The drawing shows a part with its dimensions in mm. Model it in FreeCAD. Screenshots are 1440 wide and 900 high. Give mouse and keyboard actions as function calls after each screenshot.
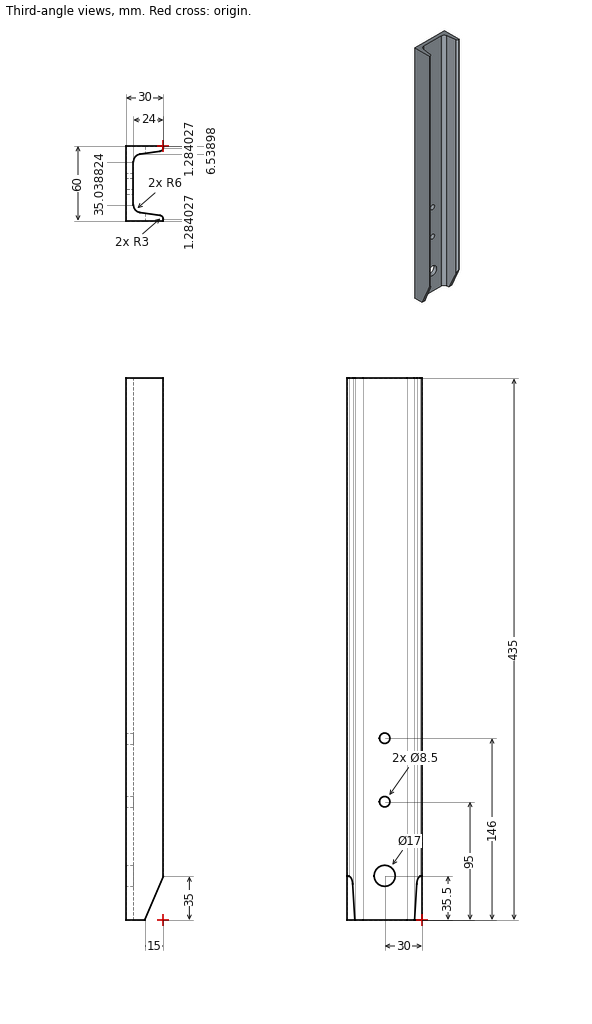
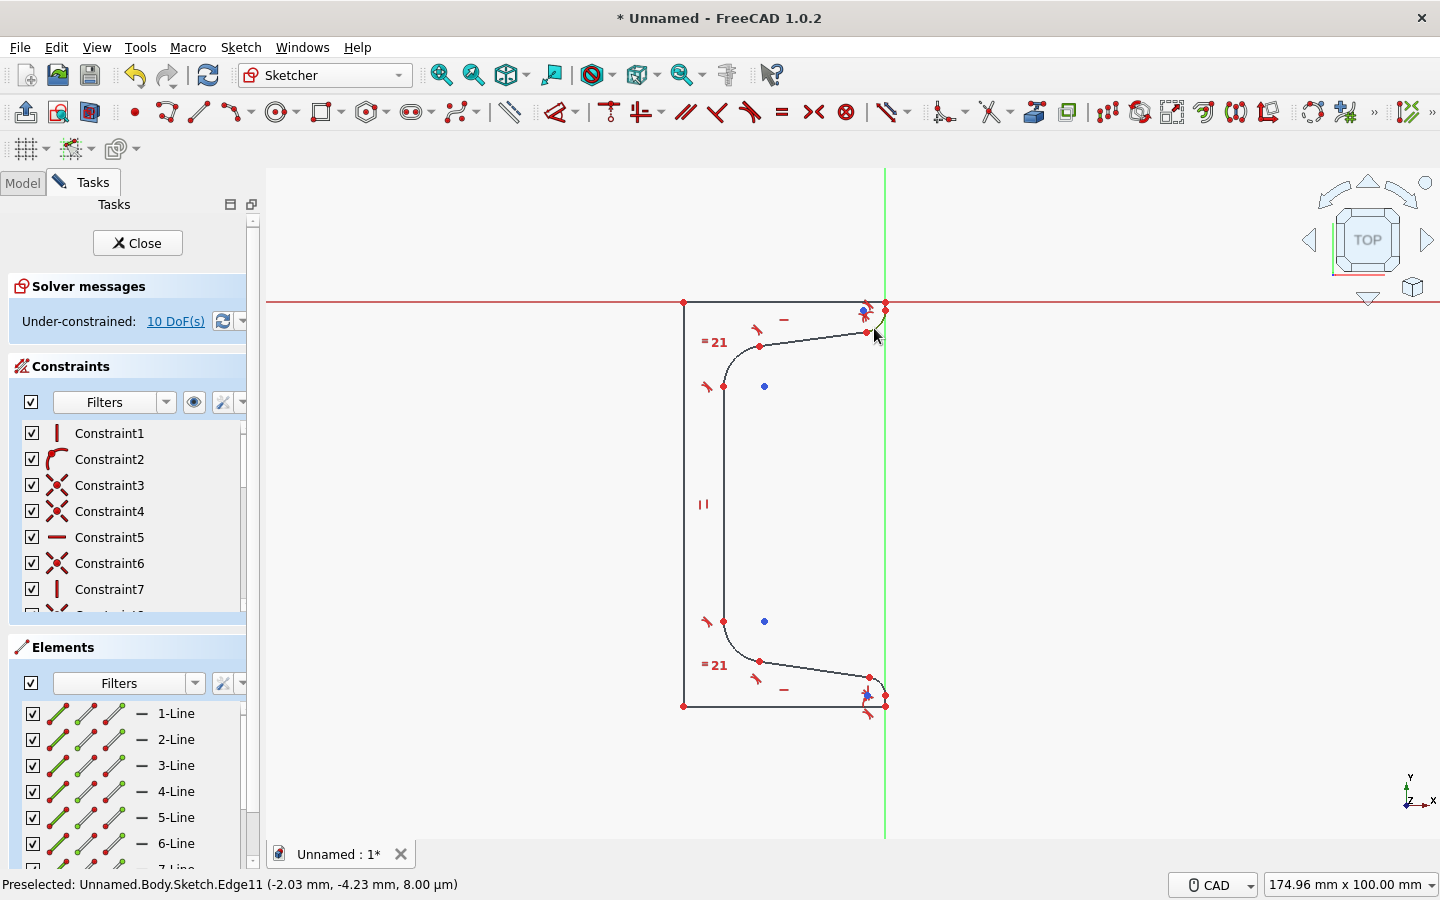
scroll(884, 688, up, 3)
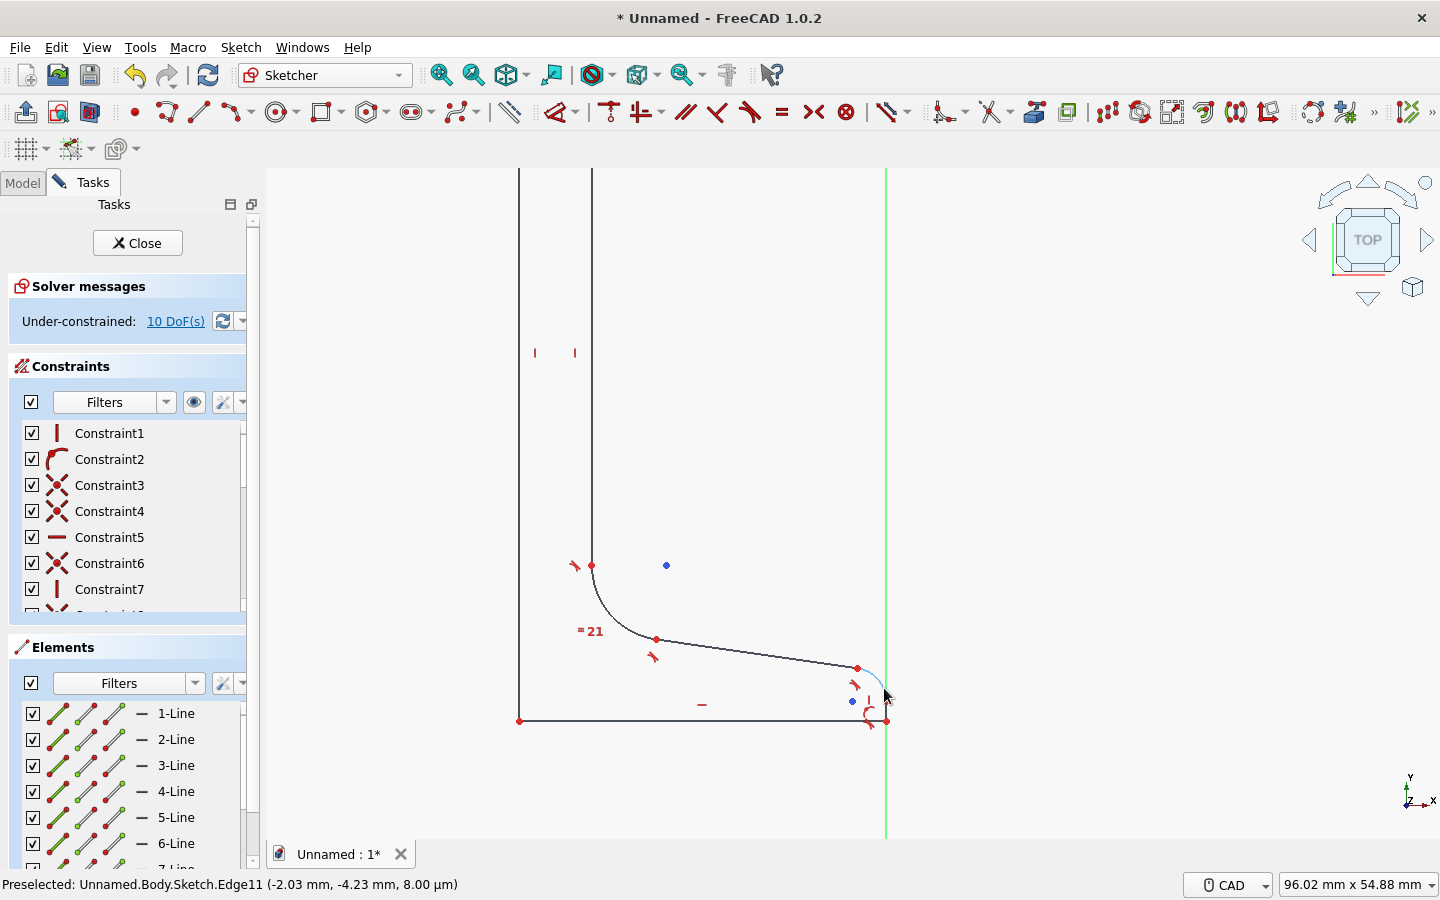
click(883, 687)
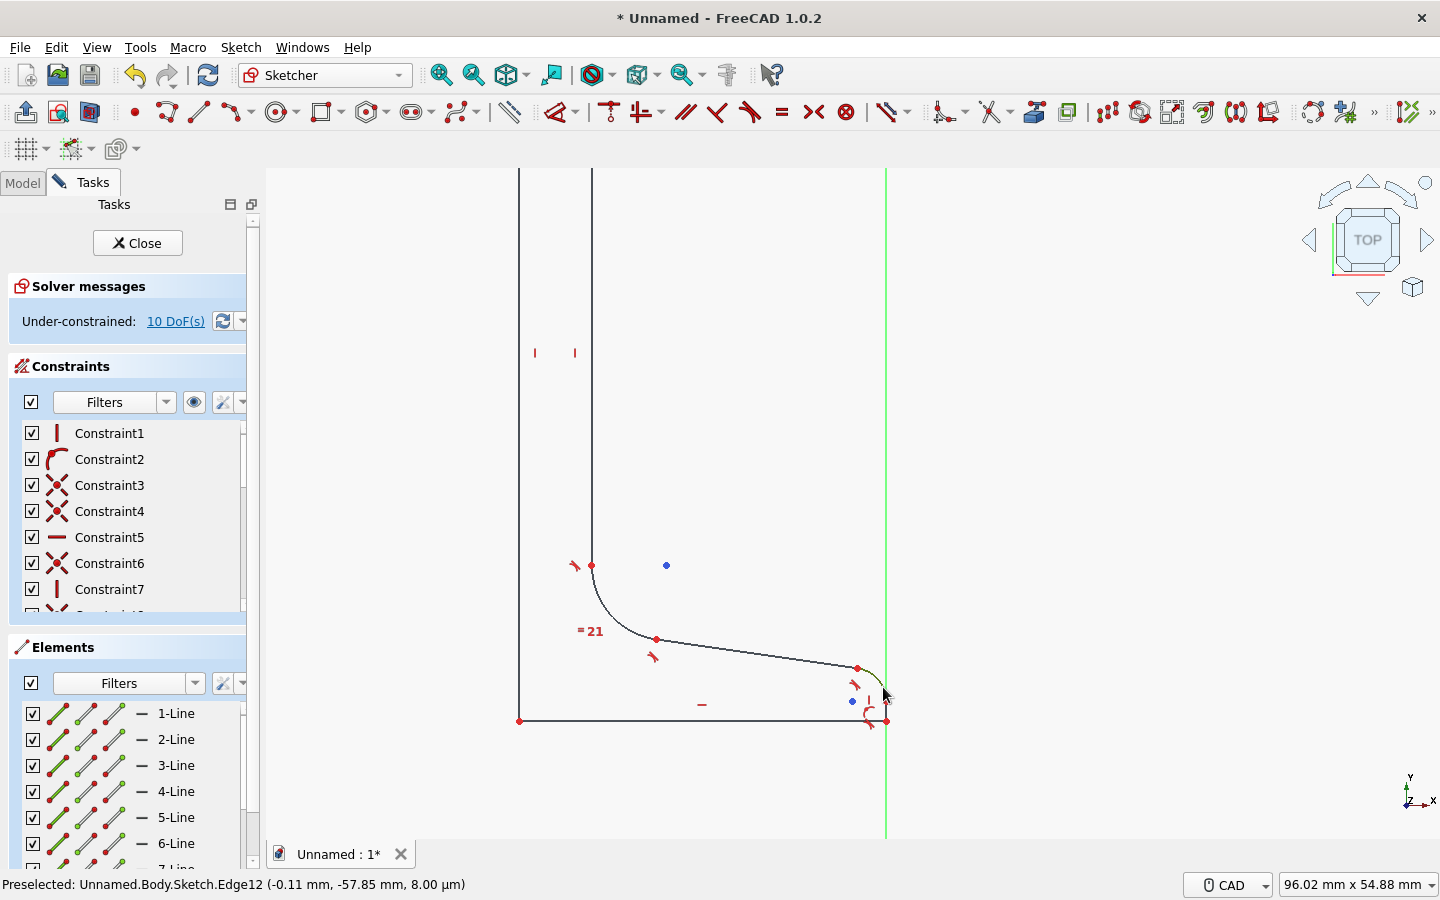
click(782, 112)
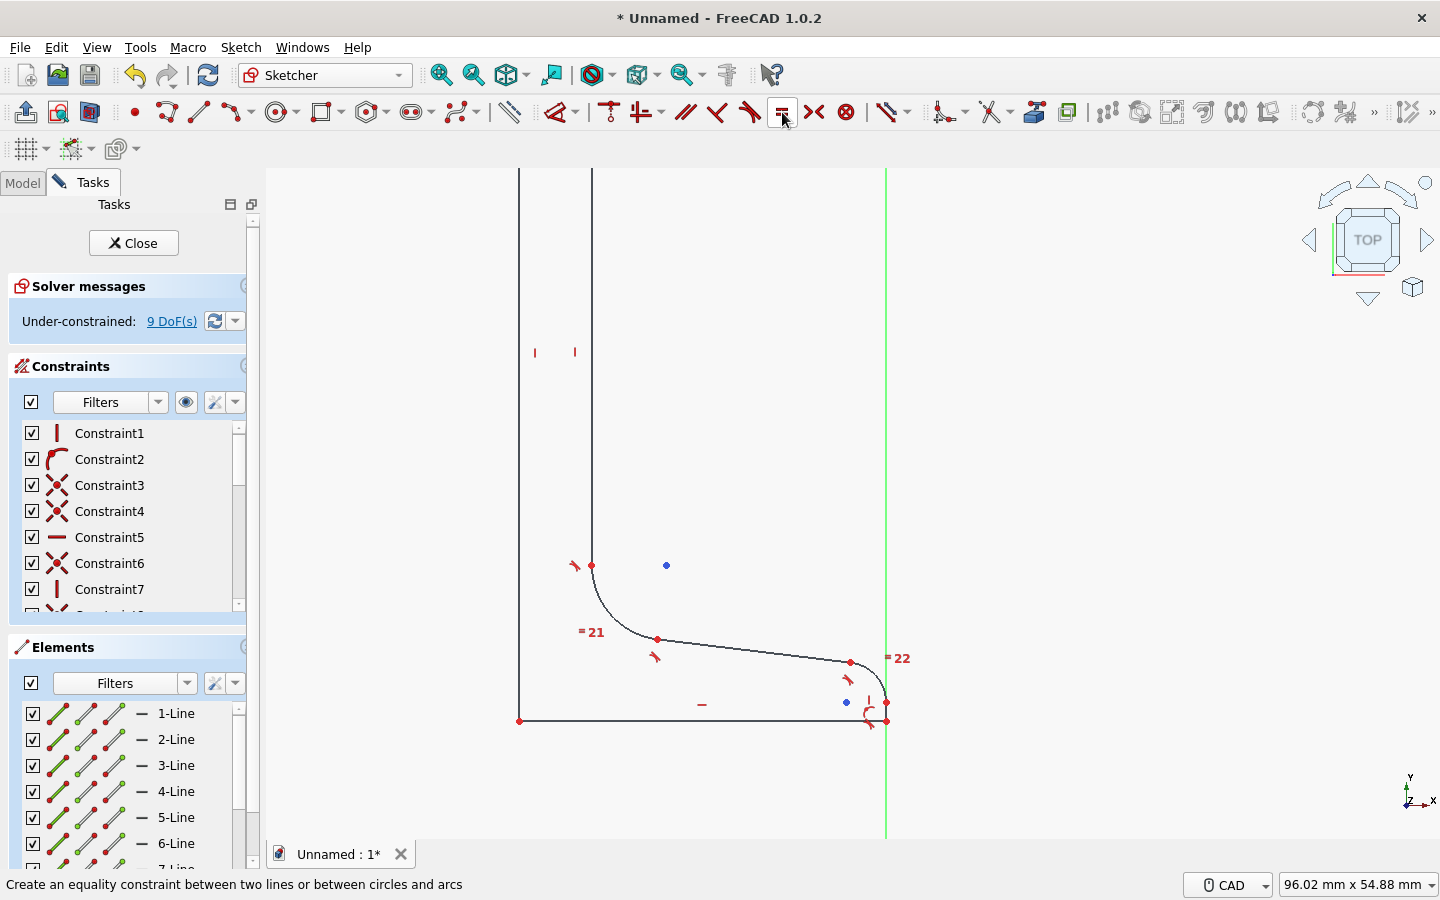
key(d)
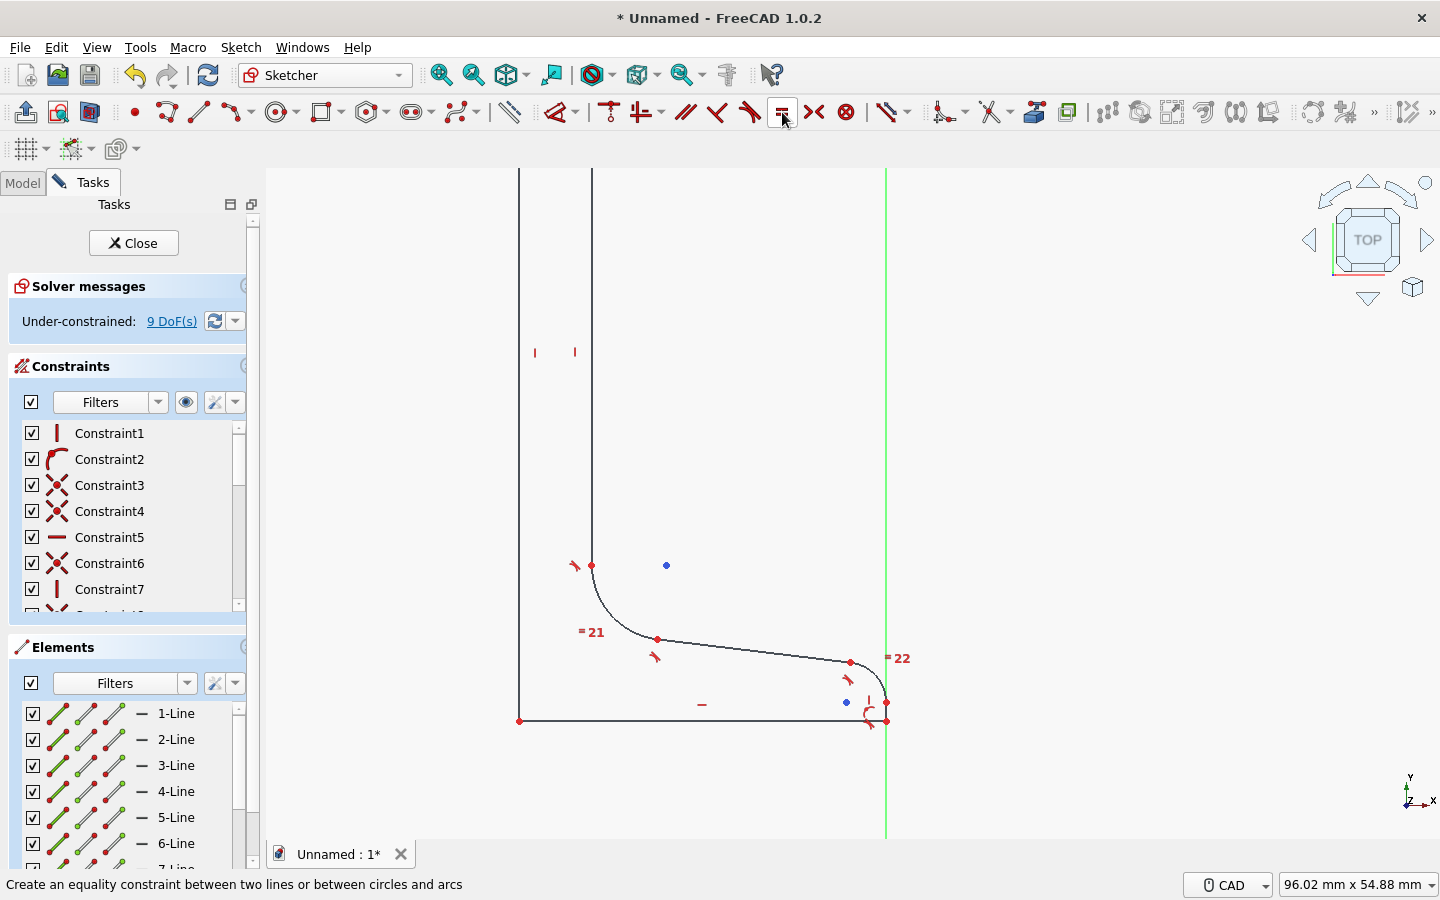
click(599, 597)
click(570, 611)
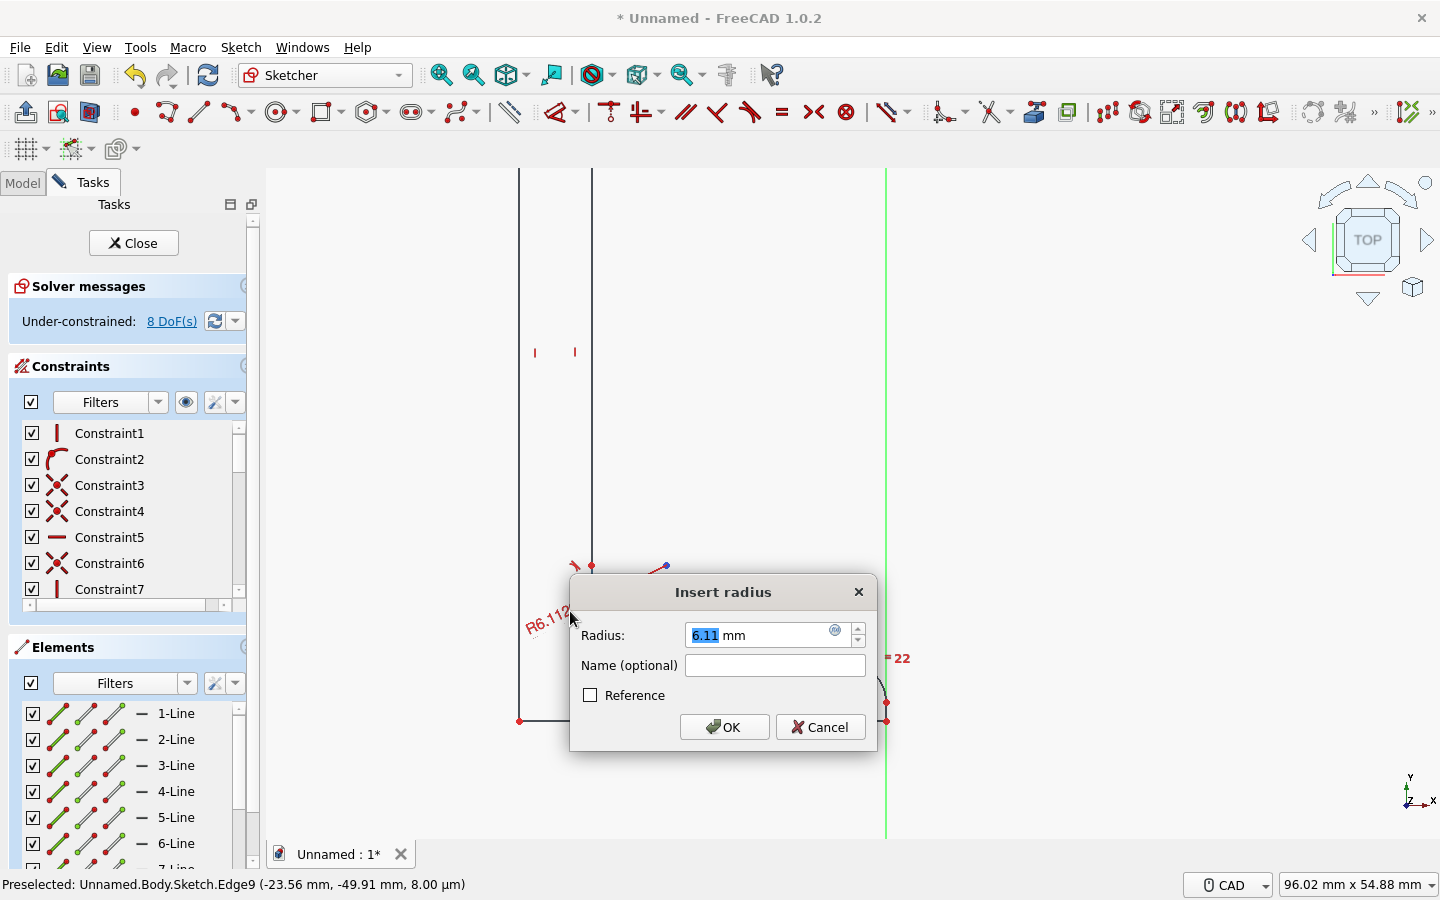
text(6)
key(Return)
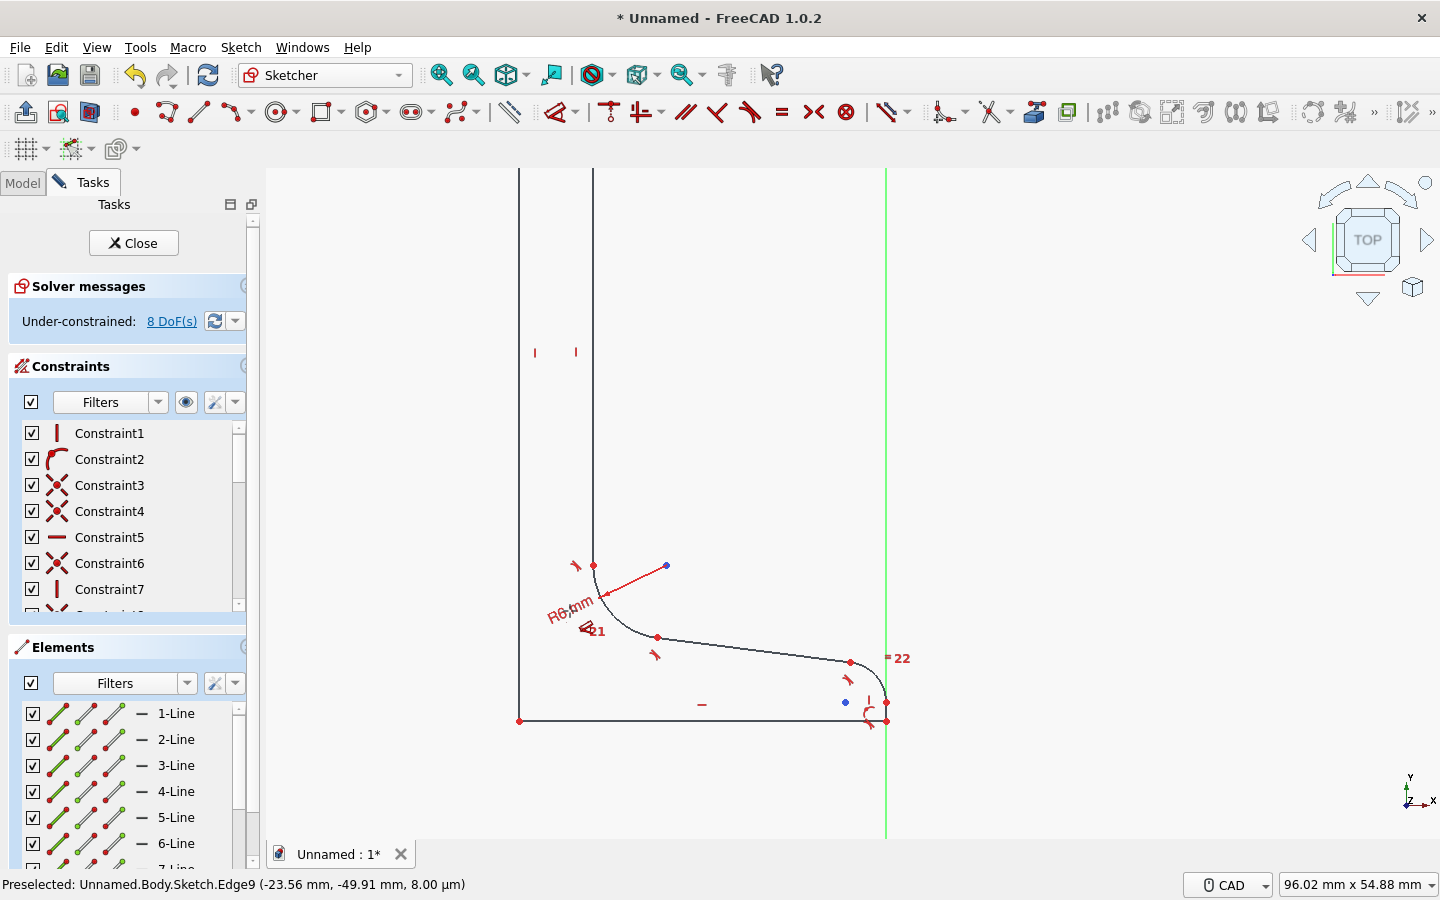
scroll(884, 689, down, 3)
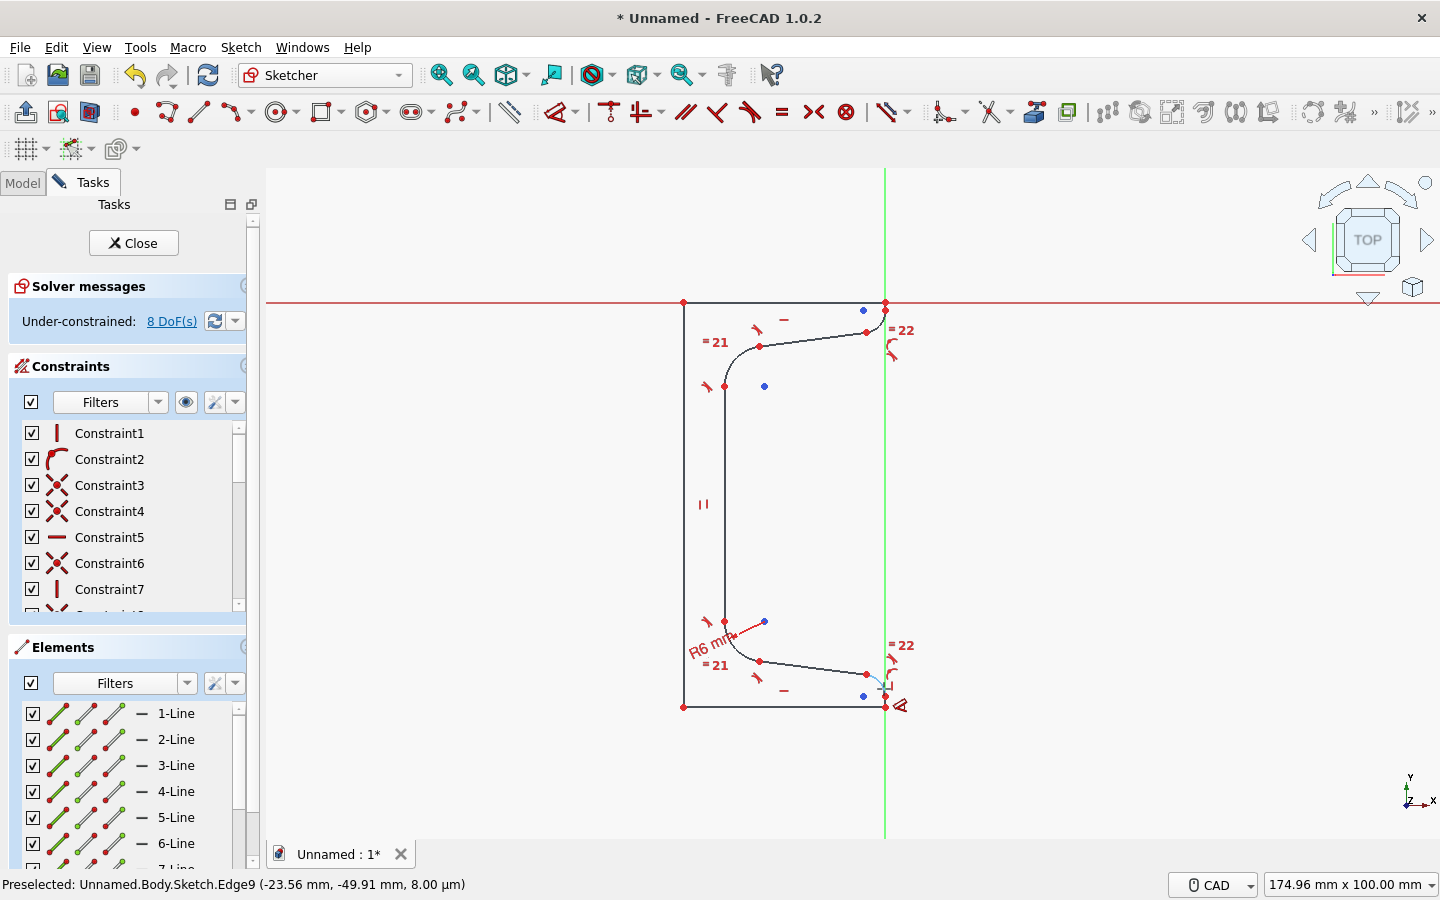
scroll(875, 330, up, 4)